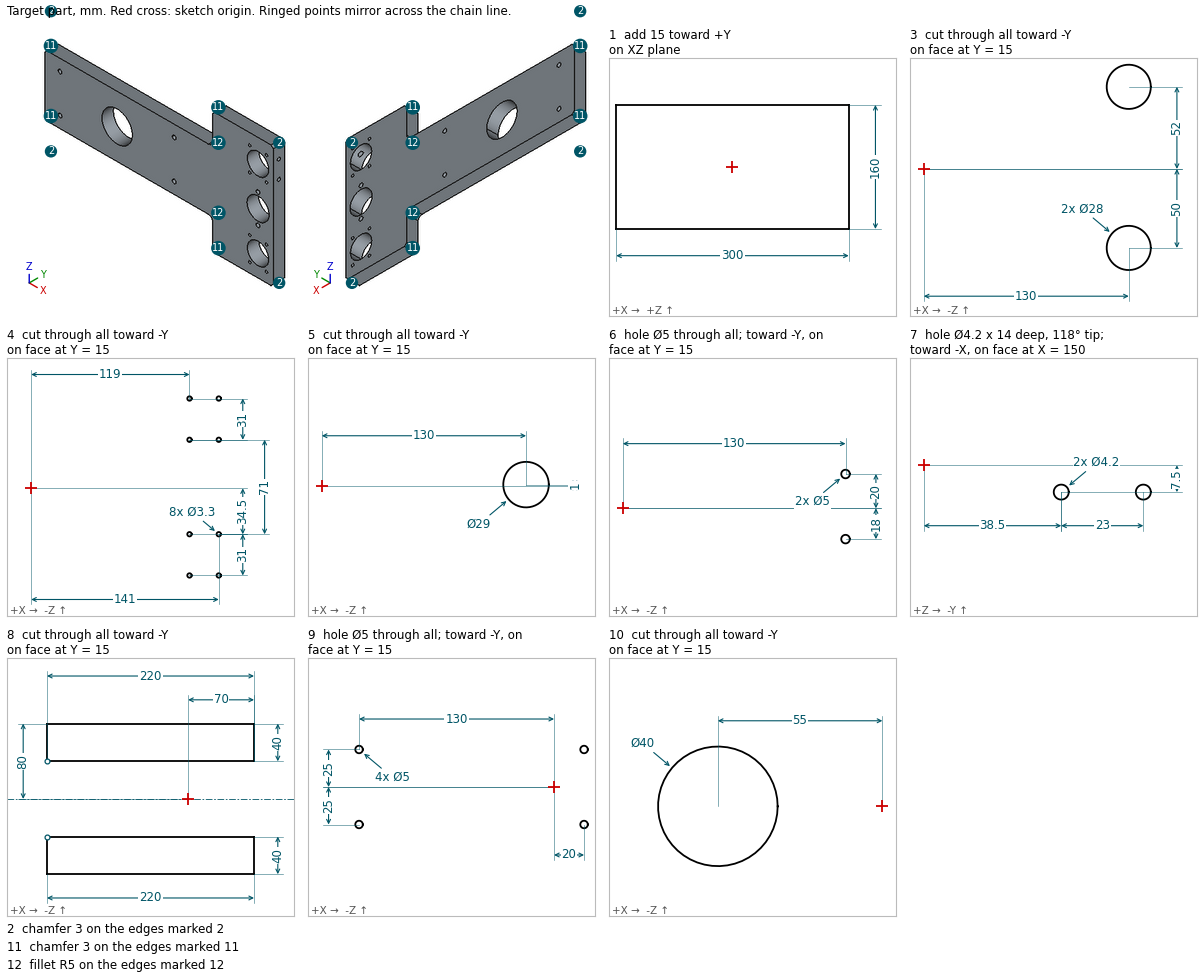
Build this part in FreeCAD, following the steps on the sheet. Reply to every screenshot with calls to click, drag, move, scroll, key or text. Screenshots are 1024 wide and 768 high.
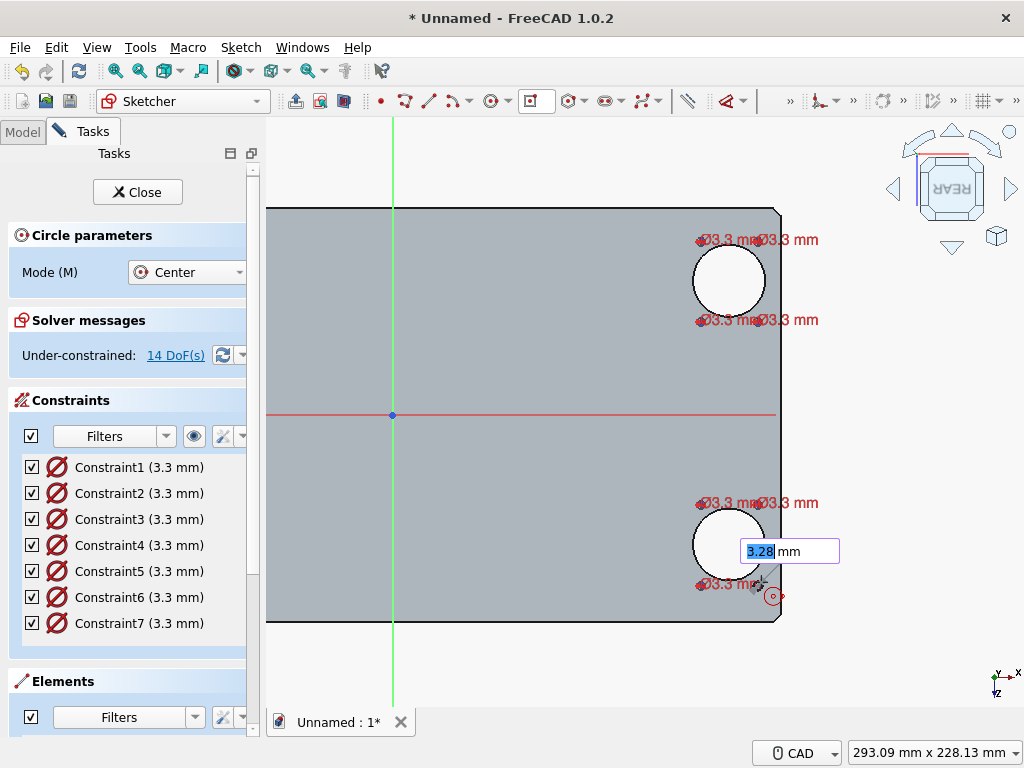
text(3.3)
key(Return)
key(Escape)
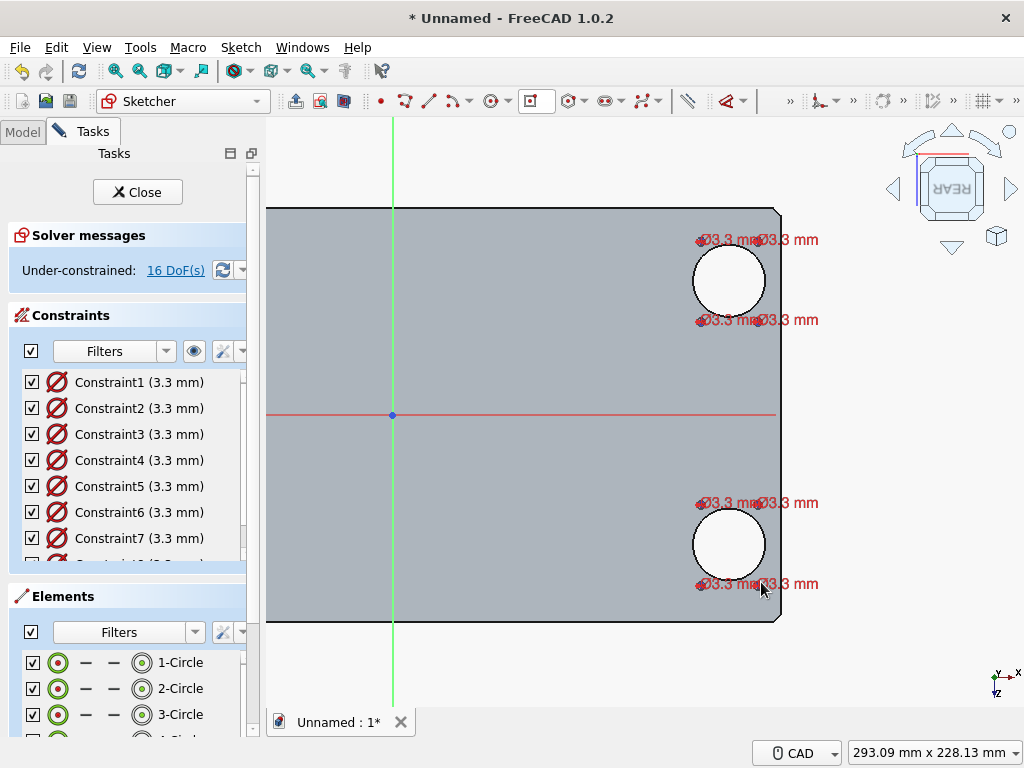
click(758, 505)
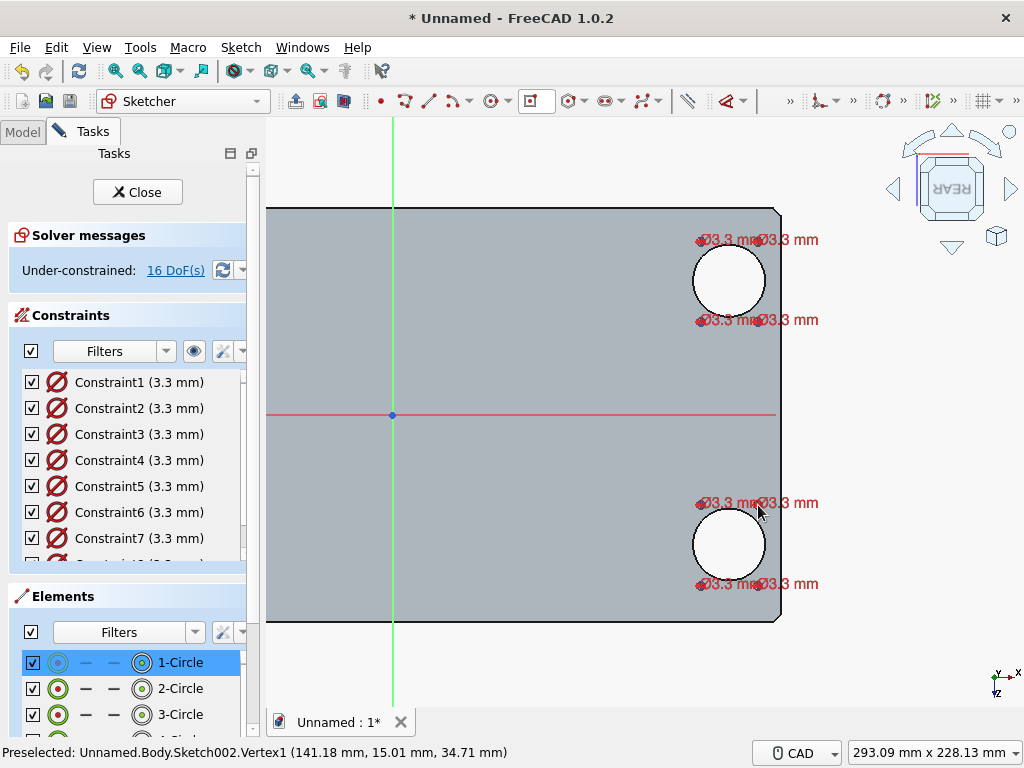
click(758, 242)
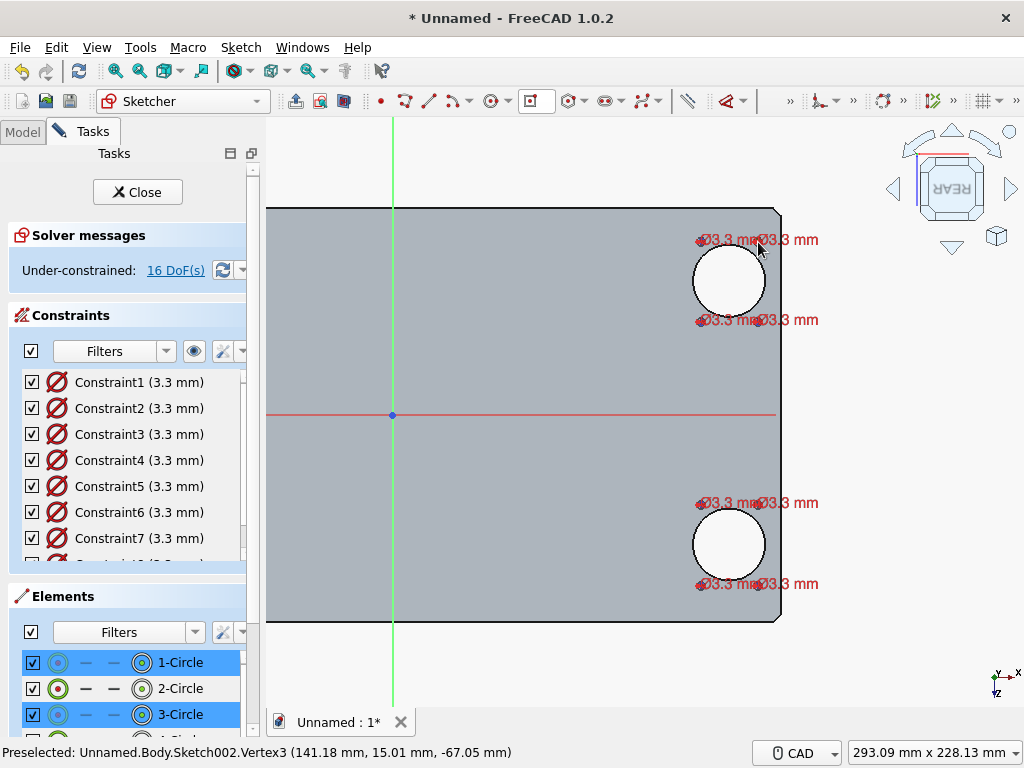
key(v)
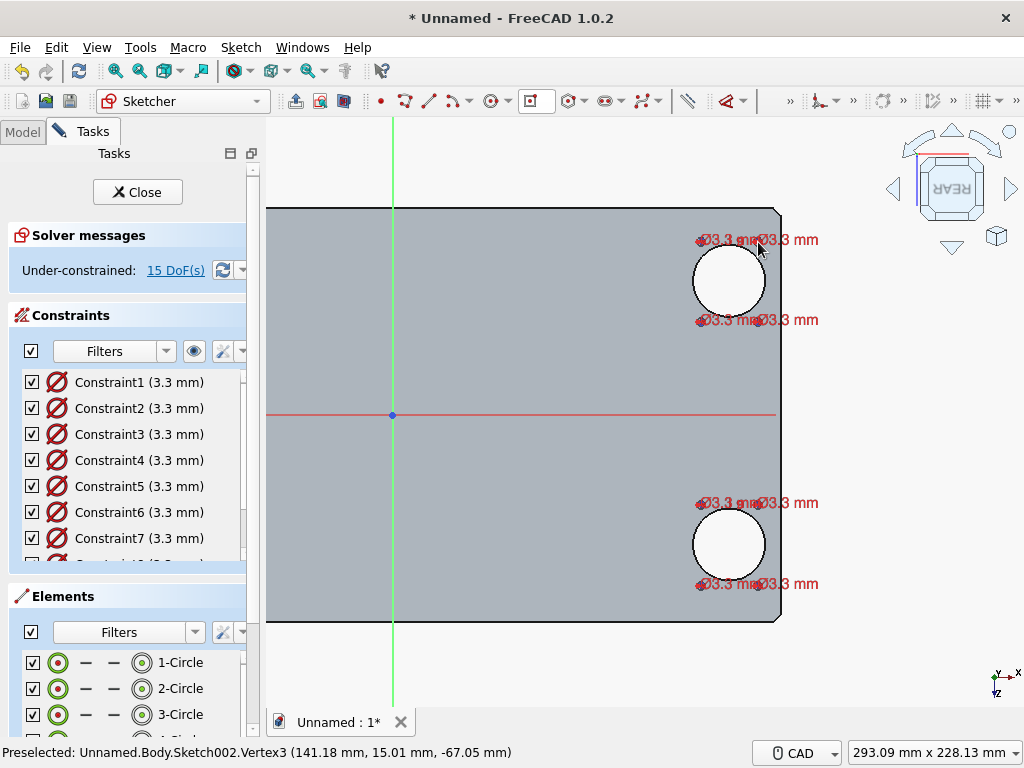
click(701, 242)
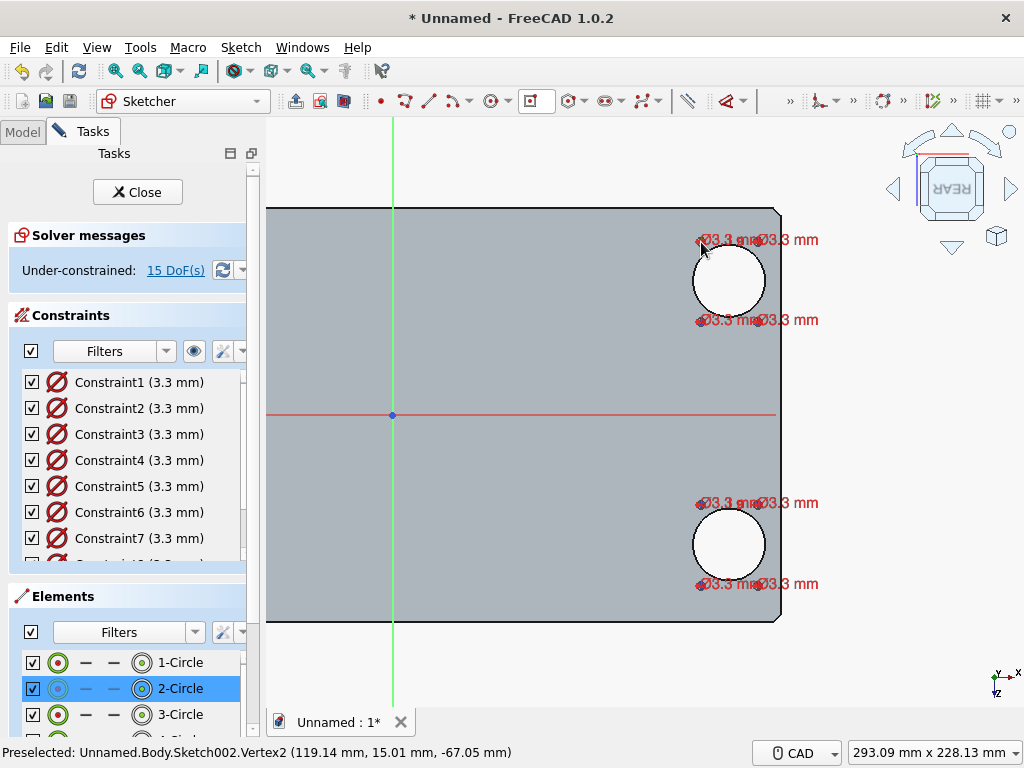
click(758, 242)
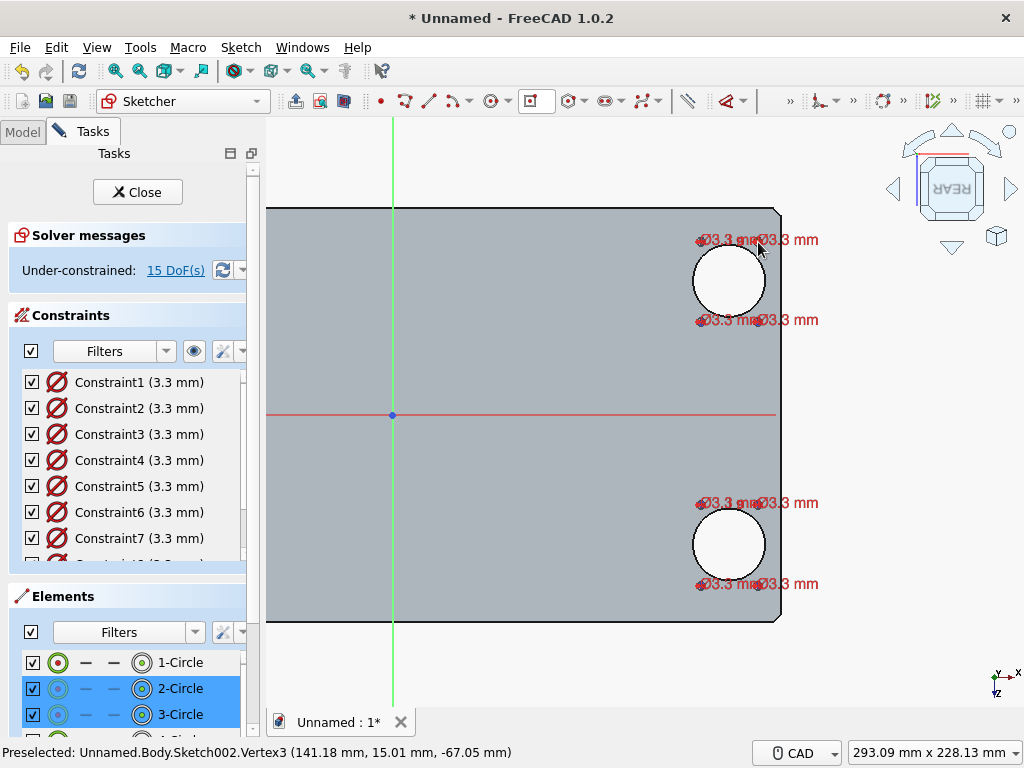
key(h)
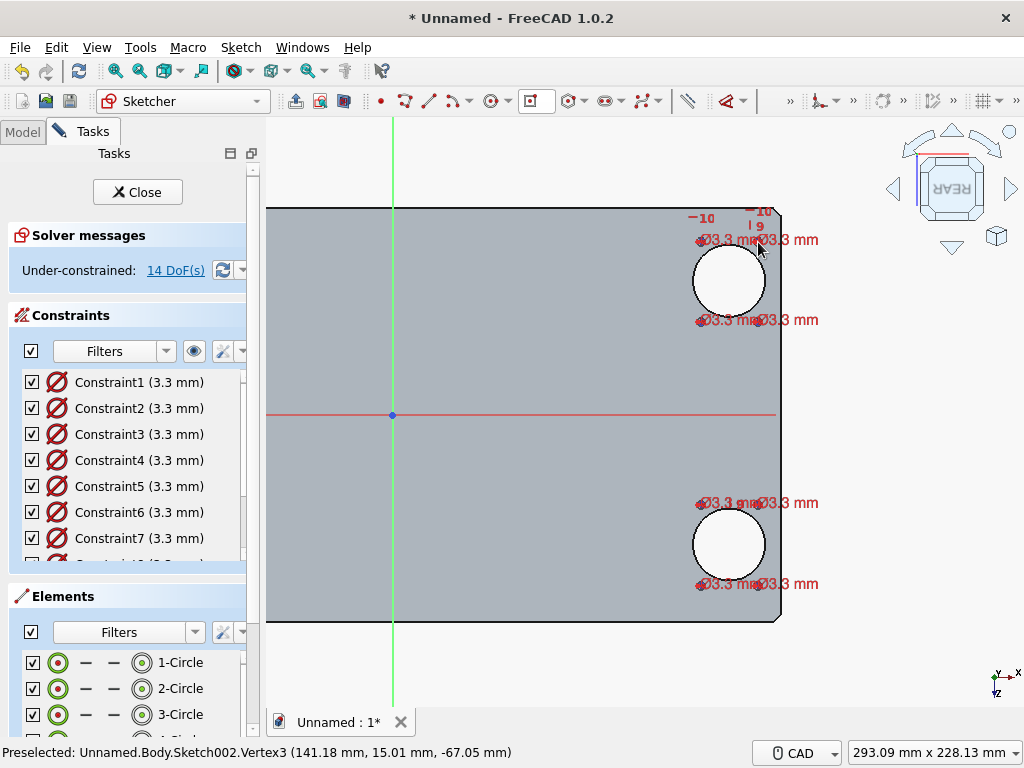
click(701, 242)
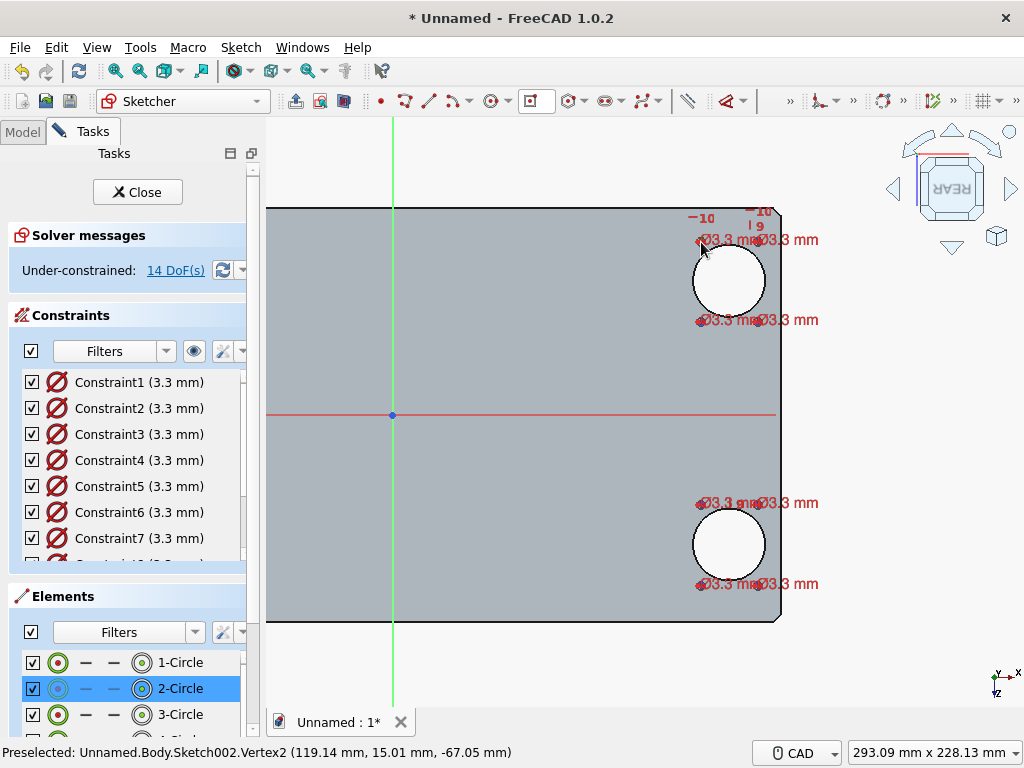
click(701, 322)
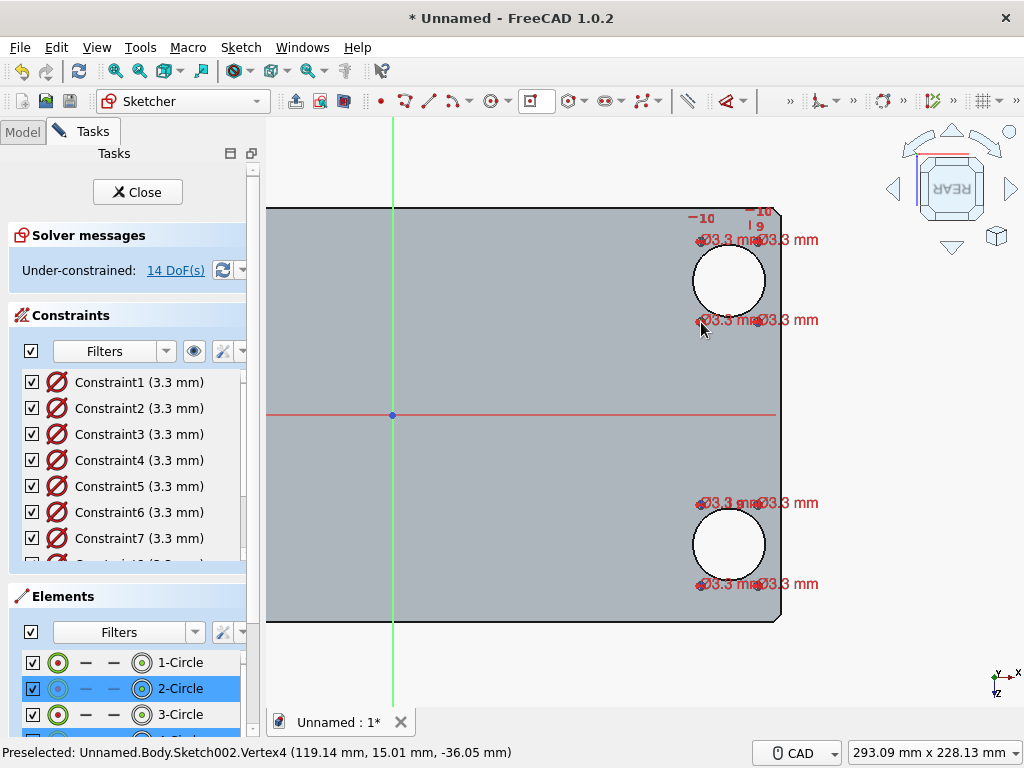
key(v)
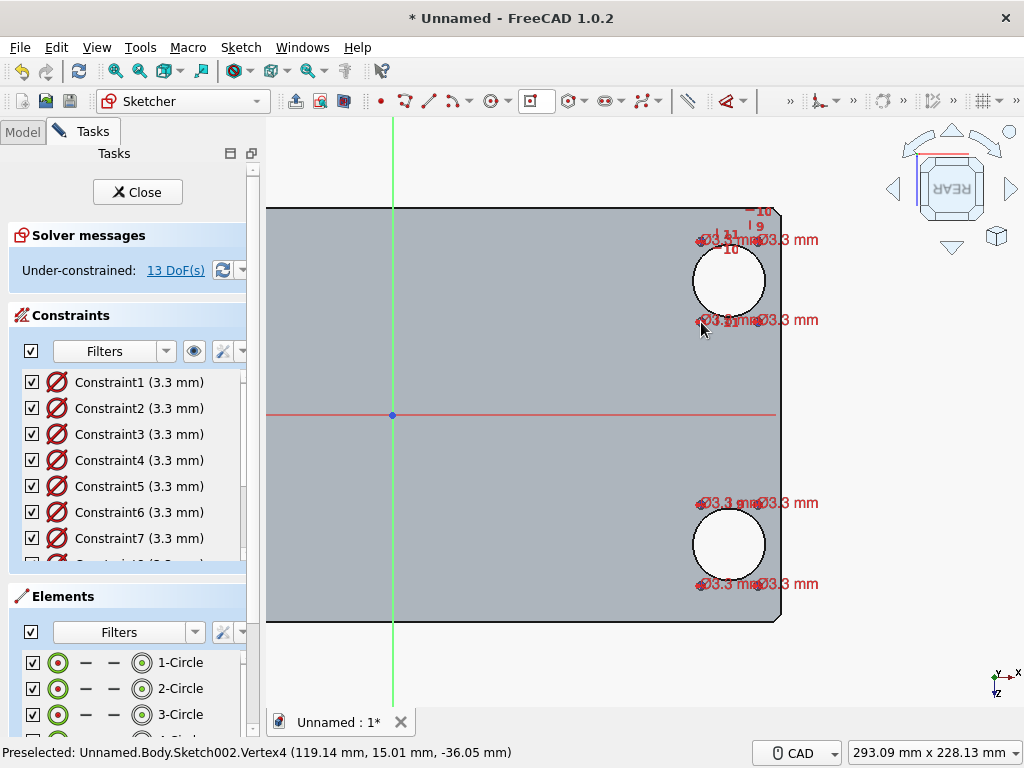
click(758, 242)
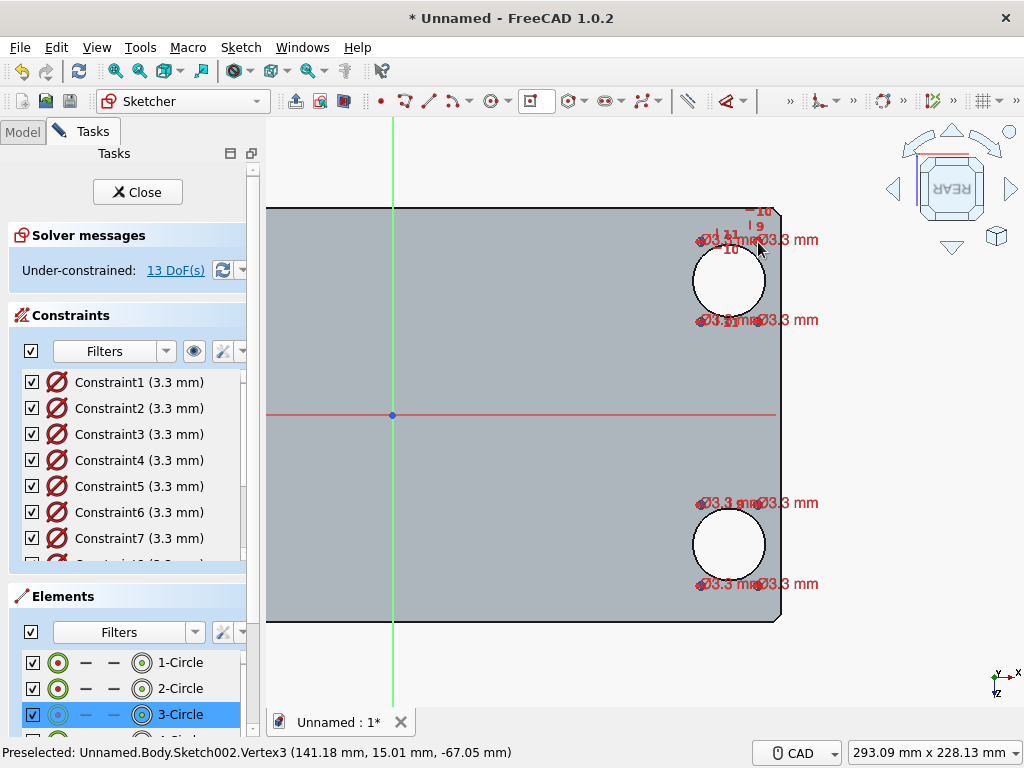
click(758, 322)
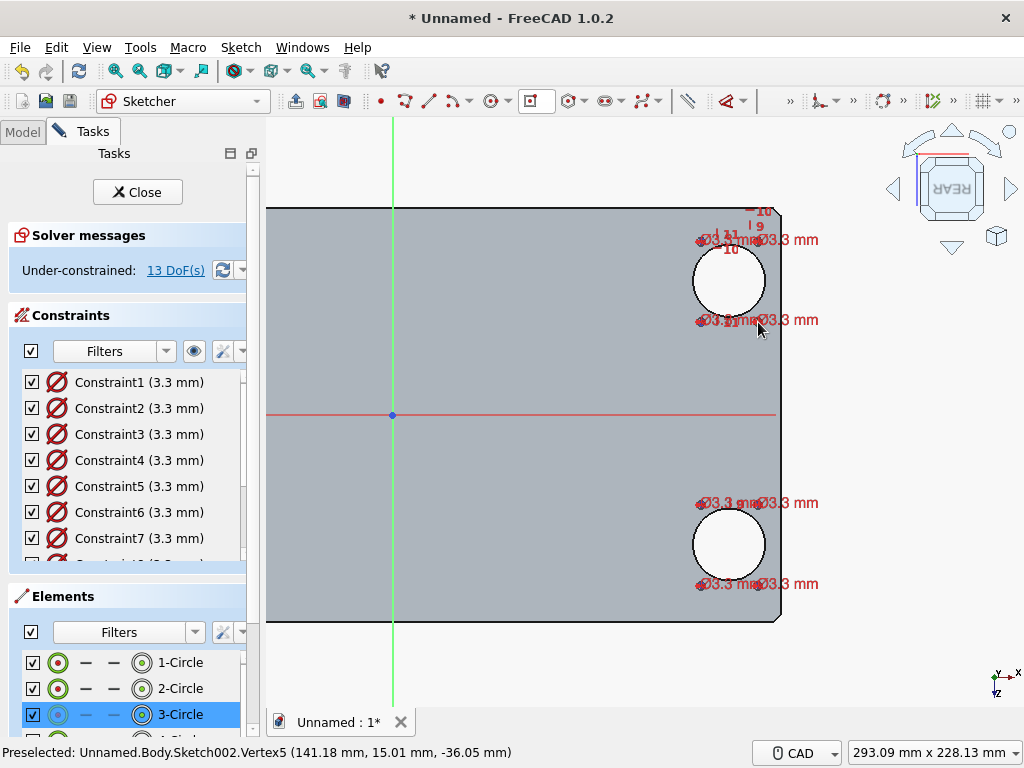
key(v)